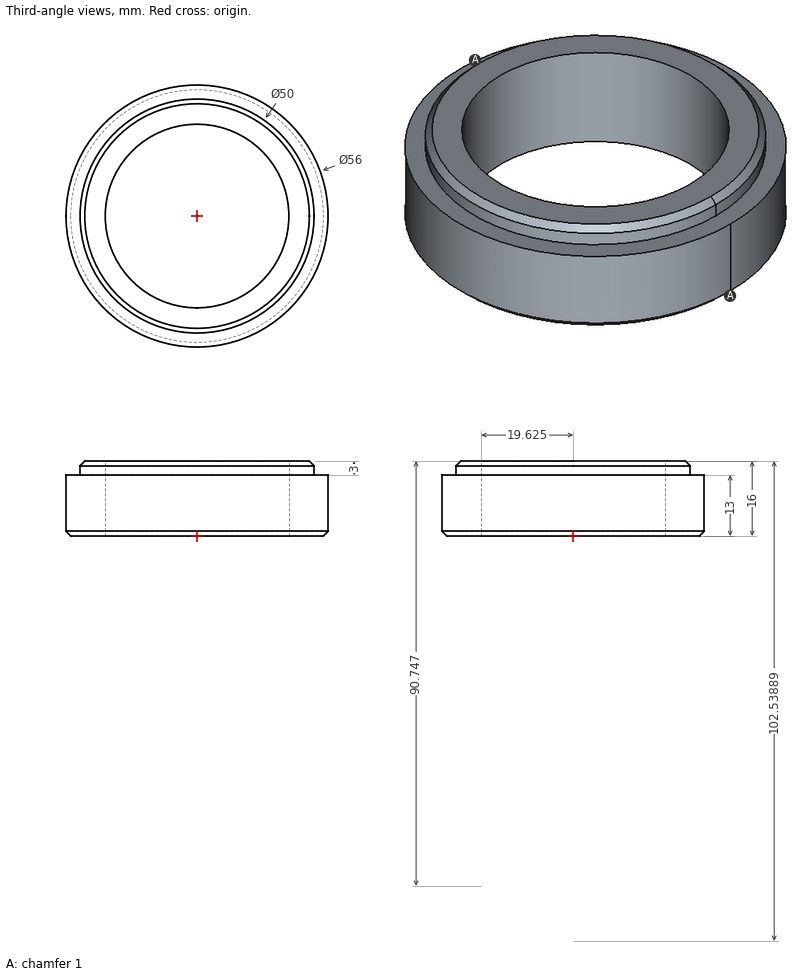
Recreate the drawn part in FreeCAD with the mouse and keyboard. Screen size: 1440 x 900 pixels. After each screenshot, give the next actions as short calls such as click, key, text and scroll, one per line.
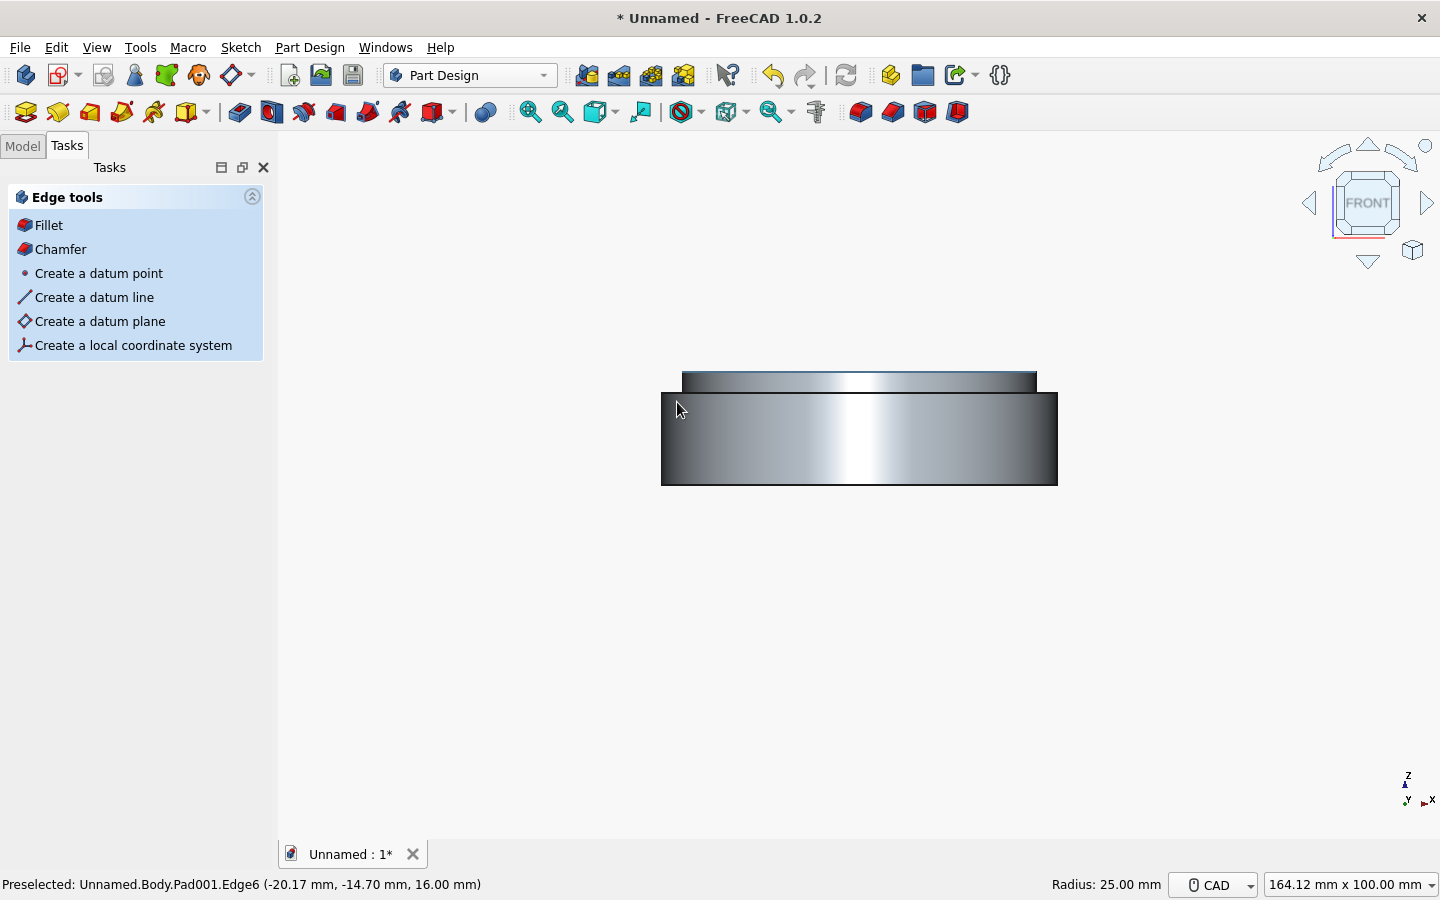
key(v)
key(f)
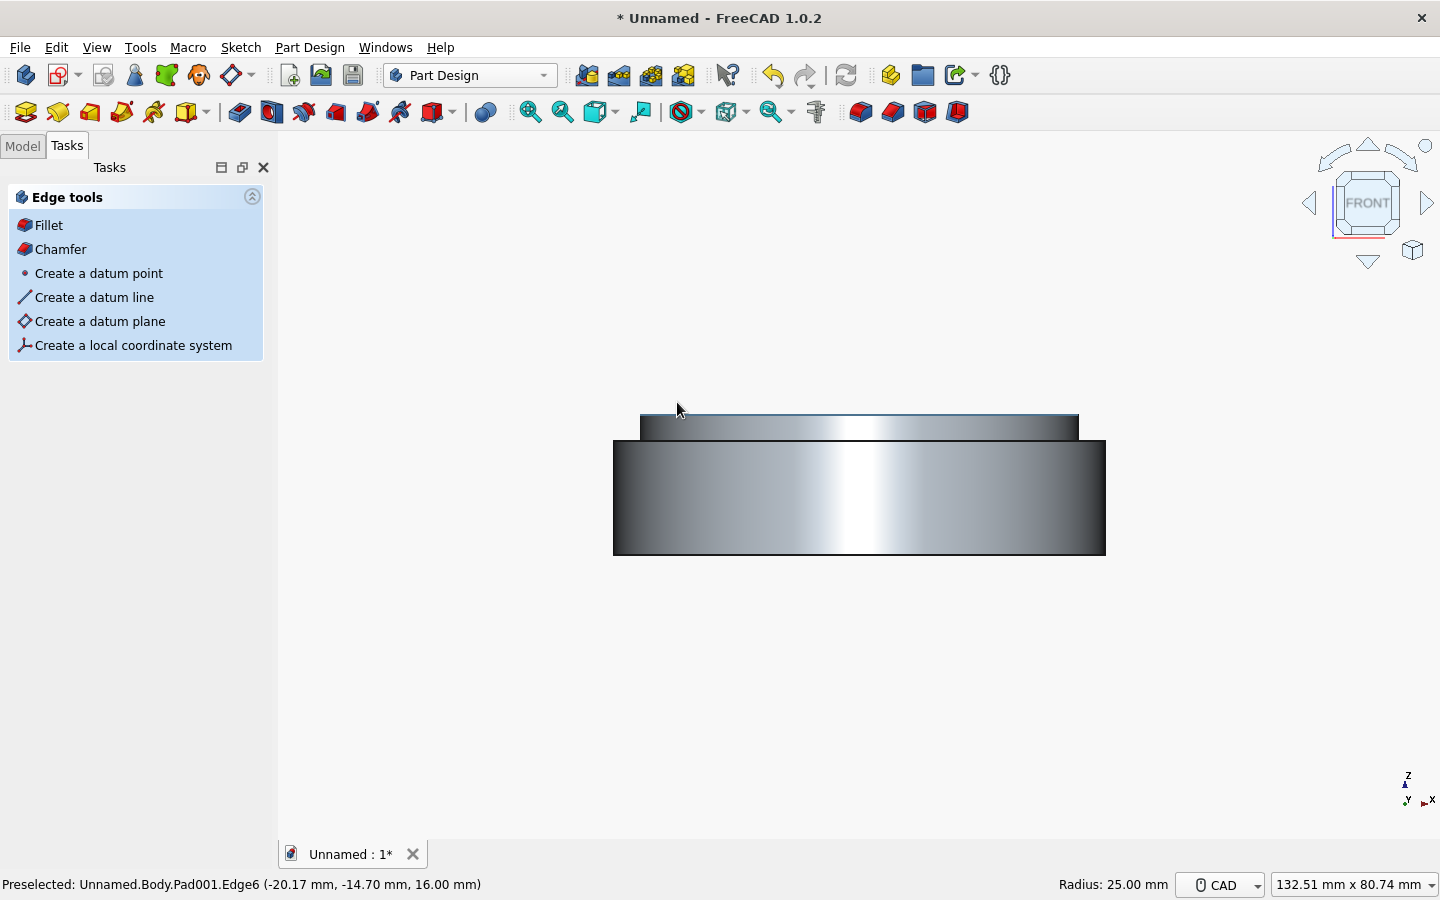
click(660, 554, ctrl)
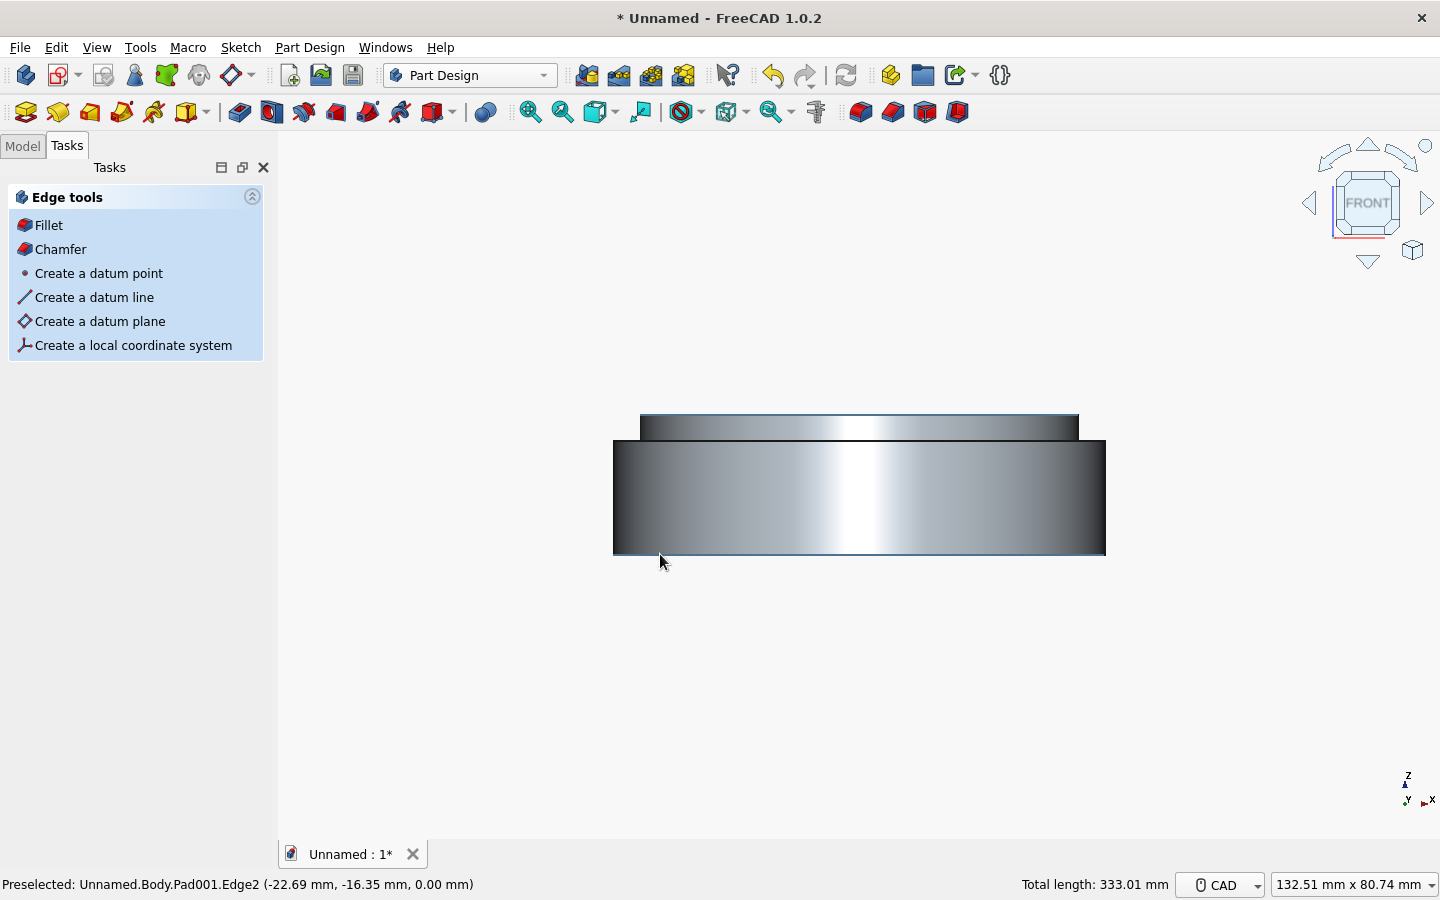
click(894, 112)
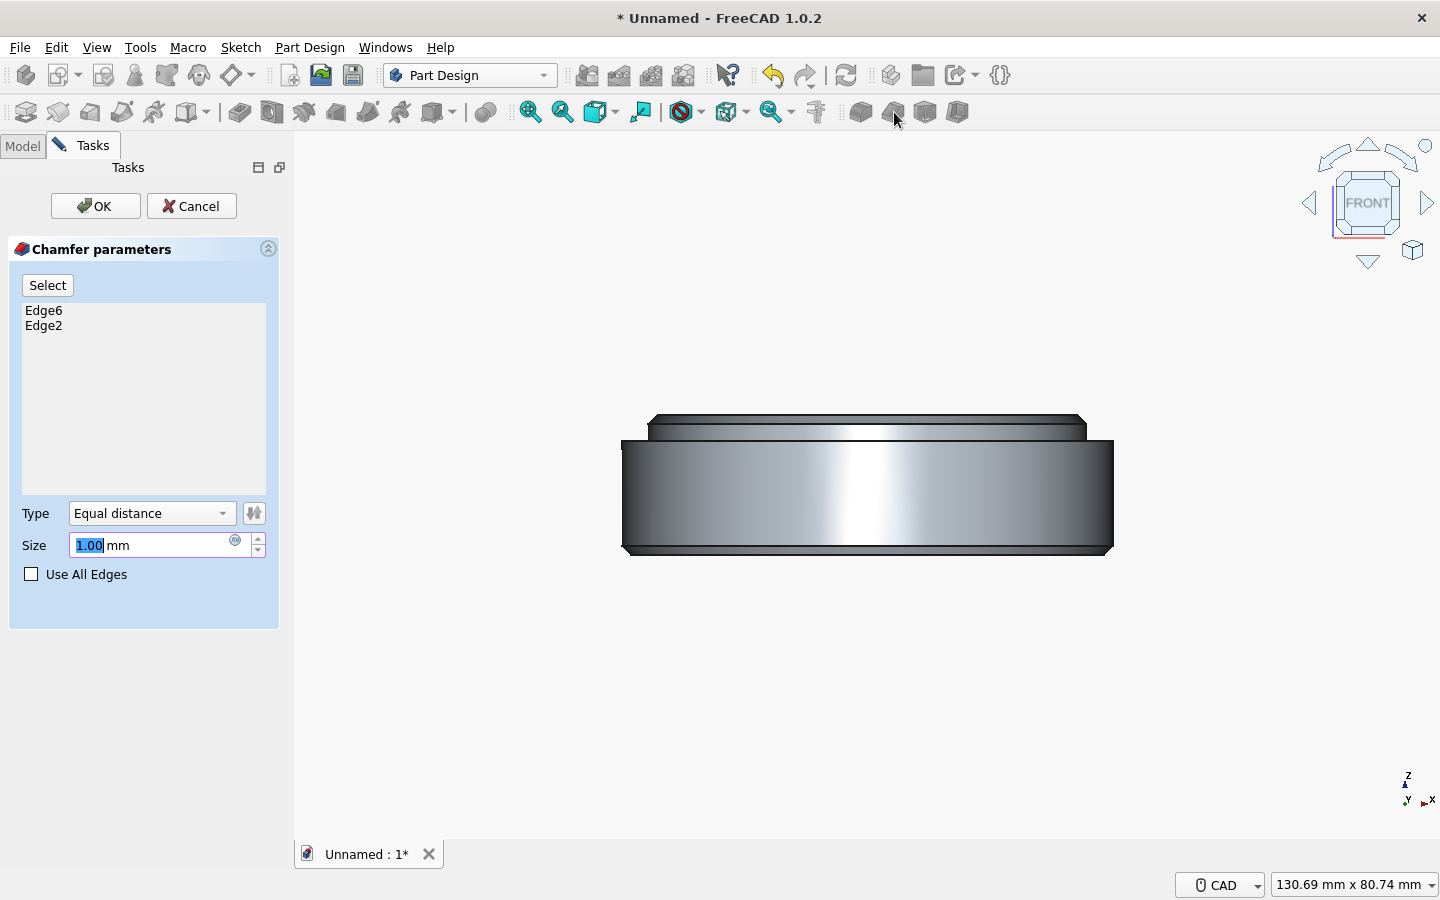
text(1)
key(Tab)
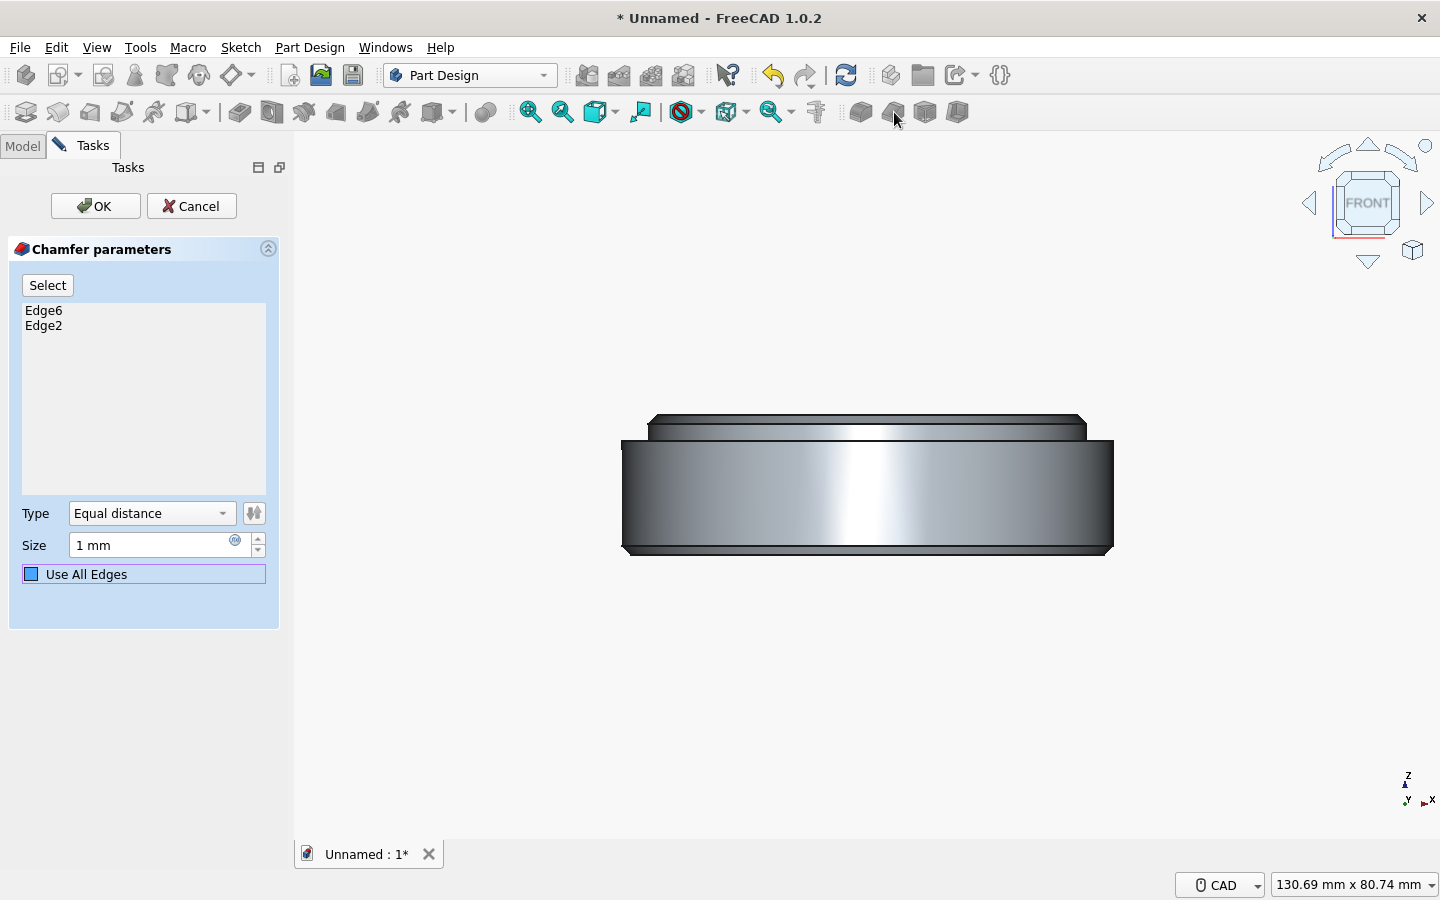
click(96, 206)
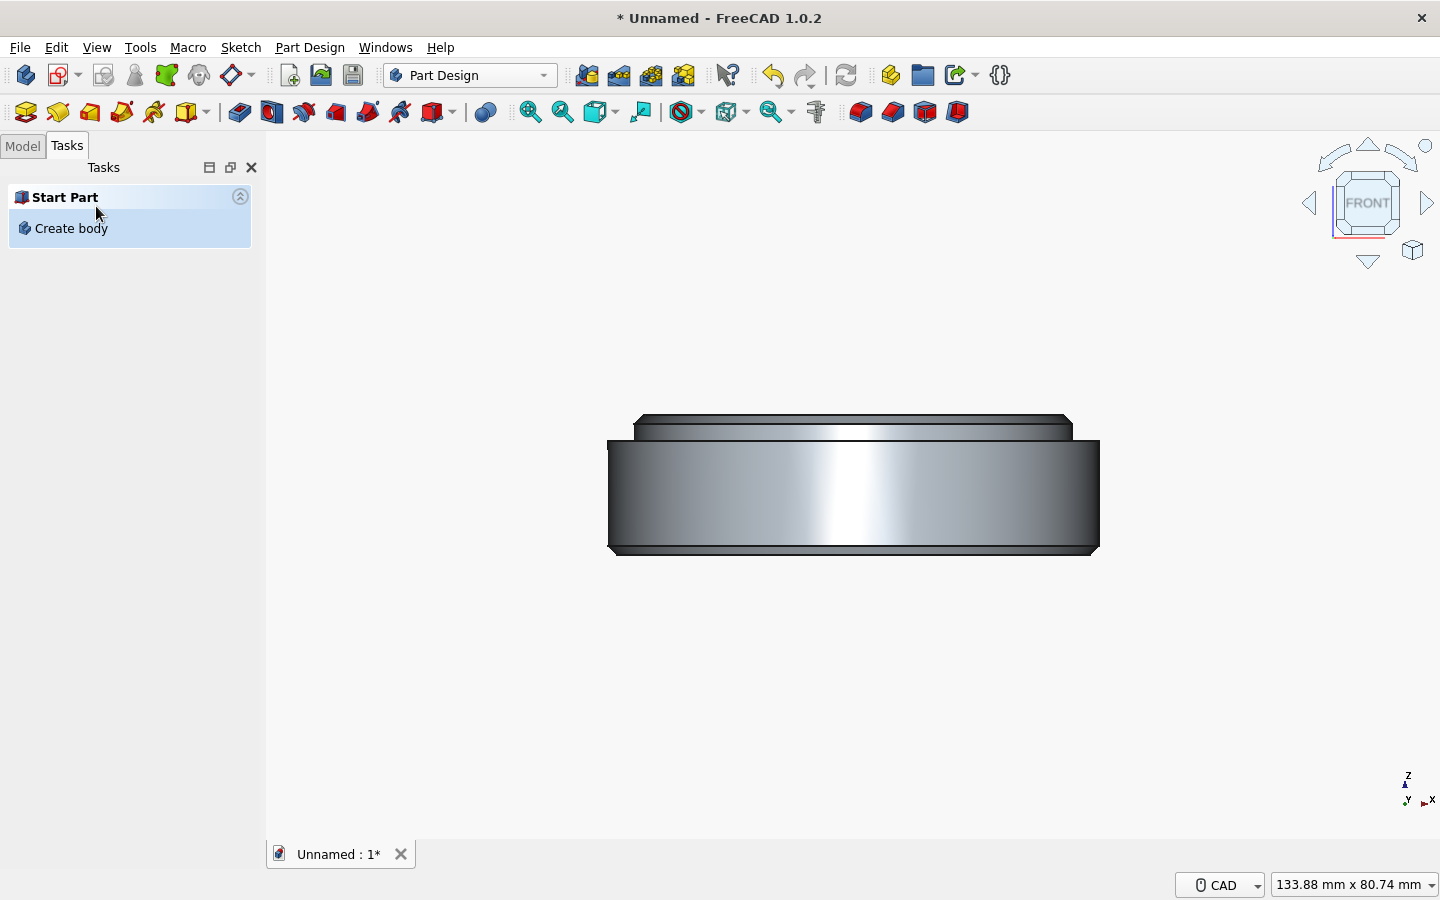
click(532, 112)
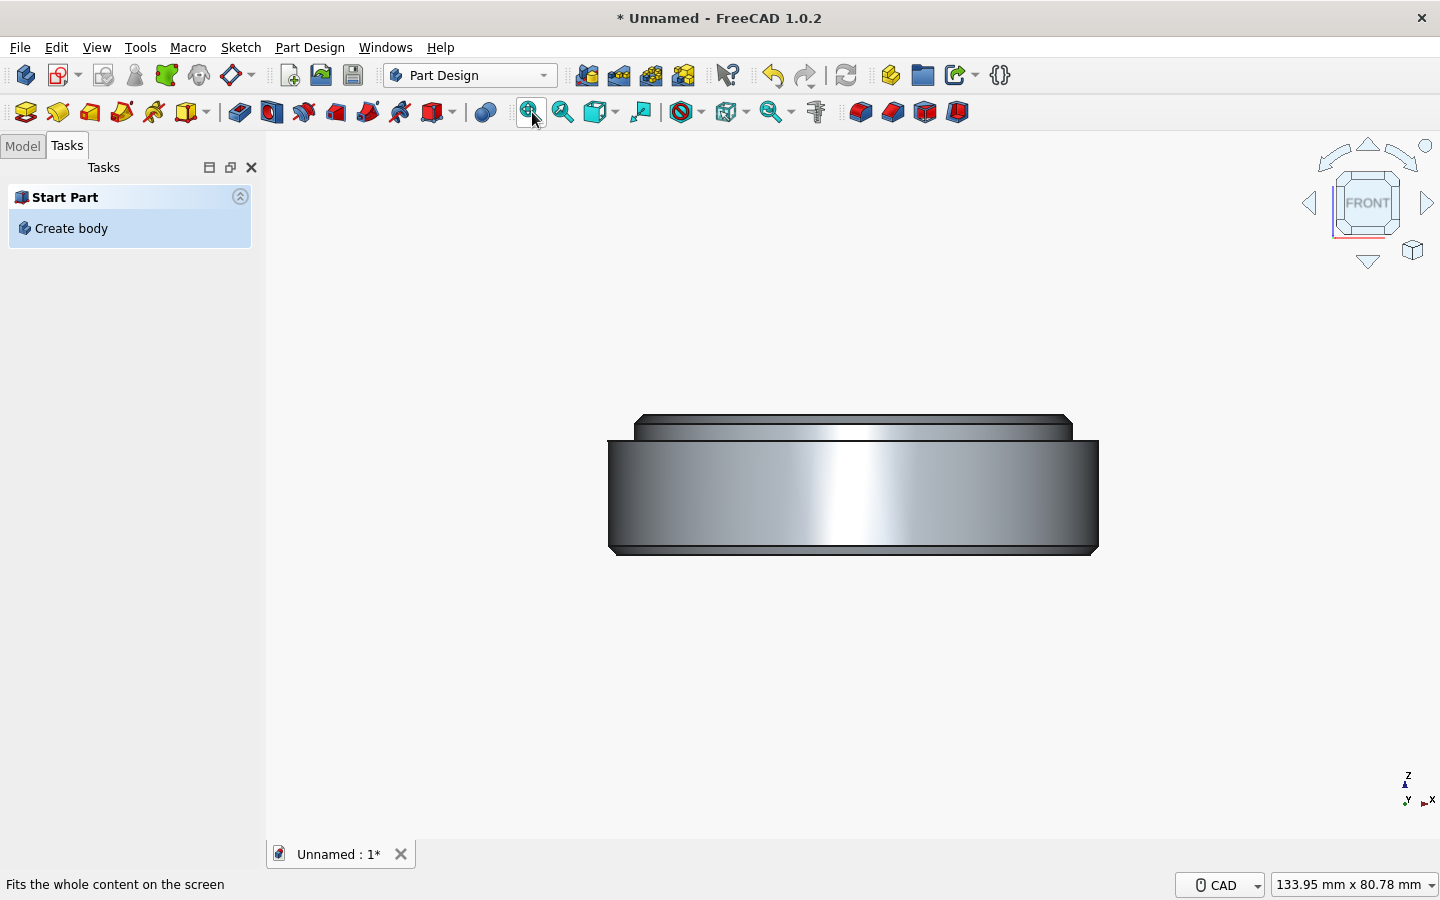
click(58, 76)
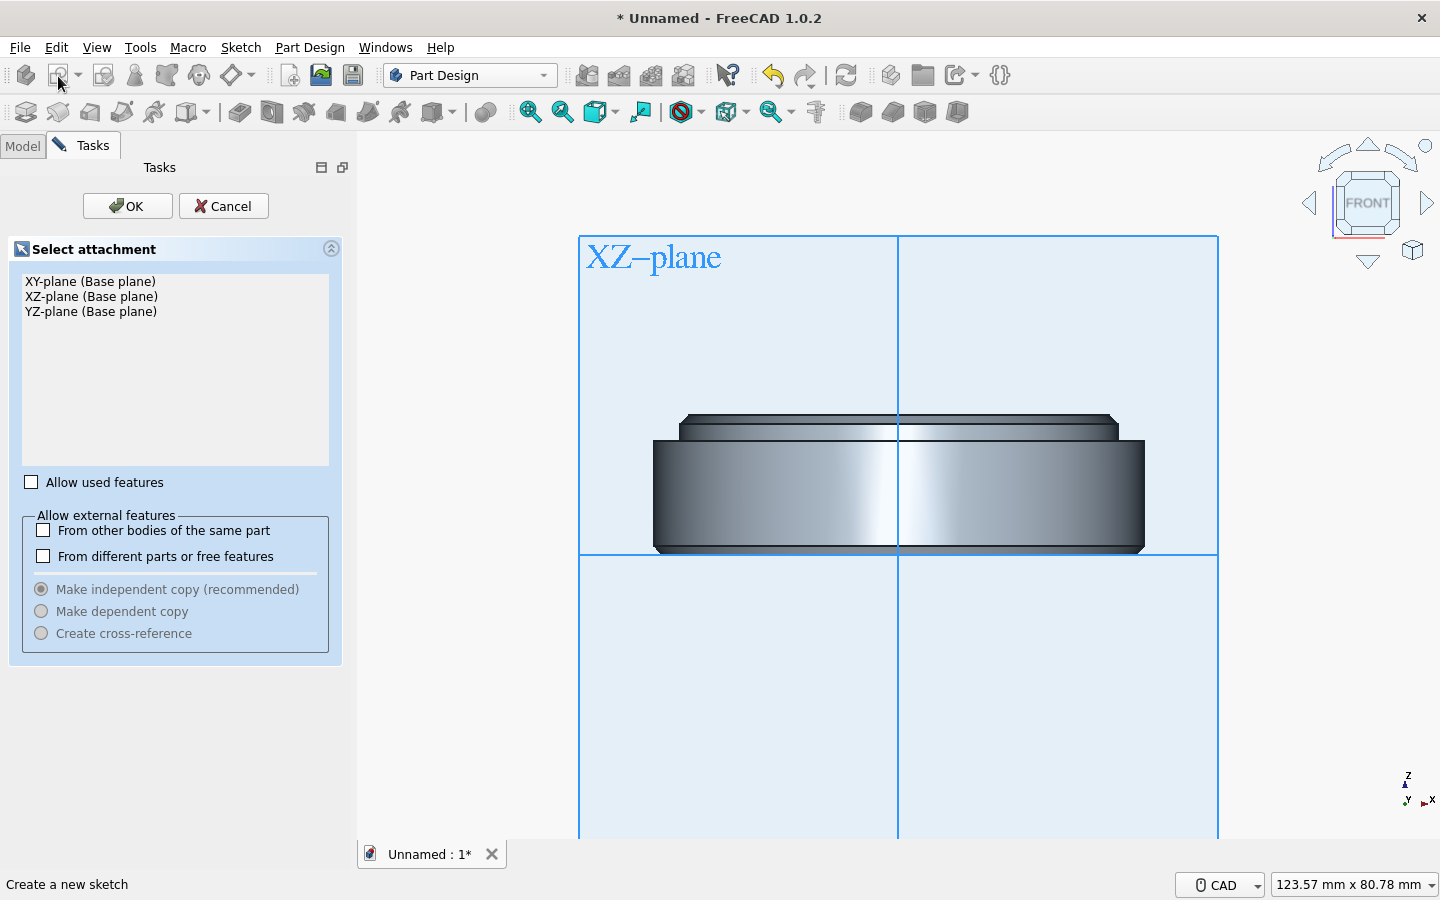
click(82, 312)